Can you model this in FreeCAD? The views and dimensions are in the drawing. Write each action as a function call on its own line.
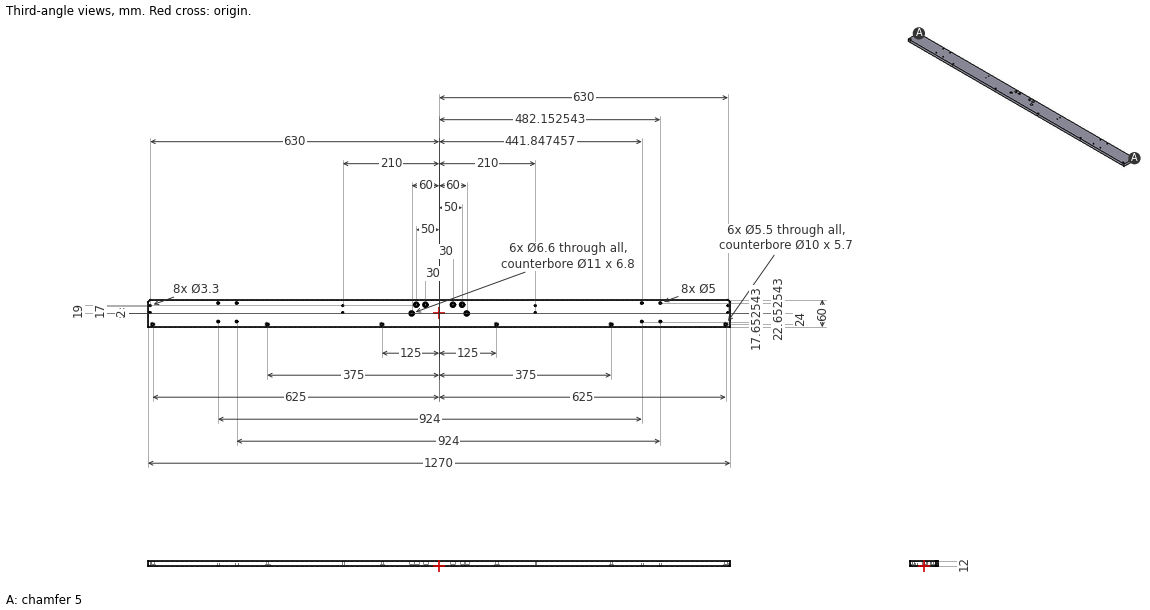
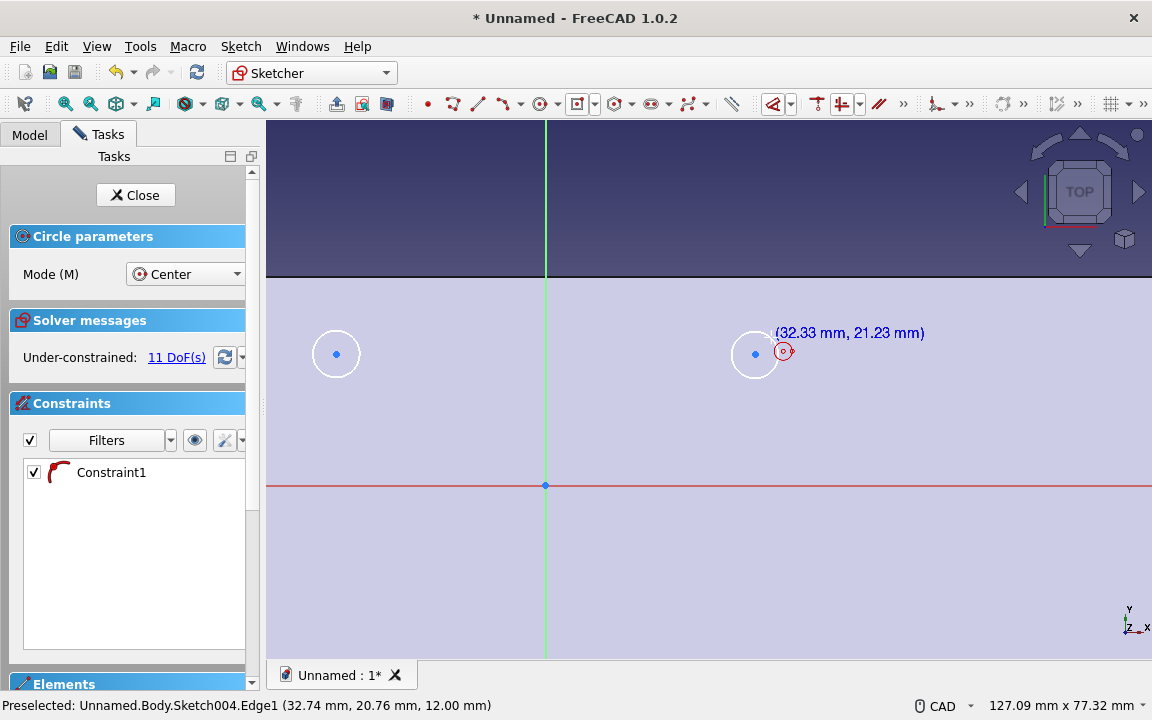
click(894, 354)
click(910, 337)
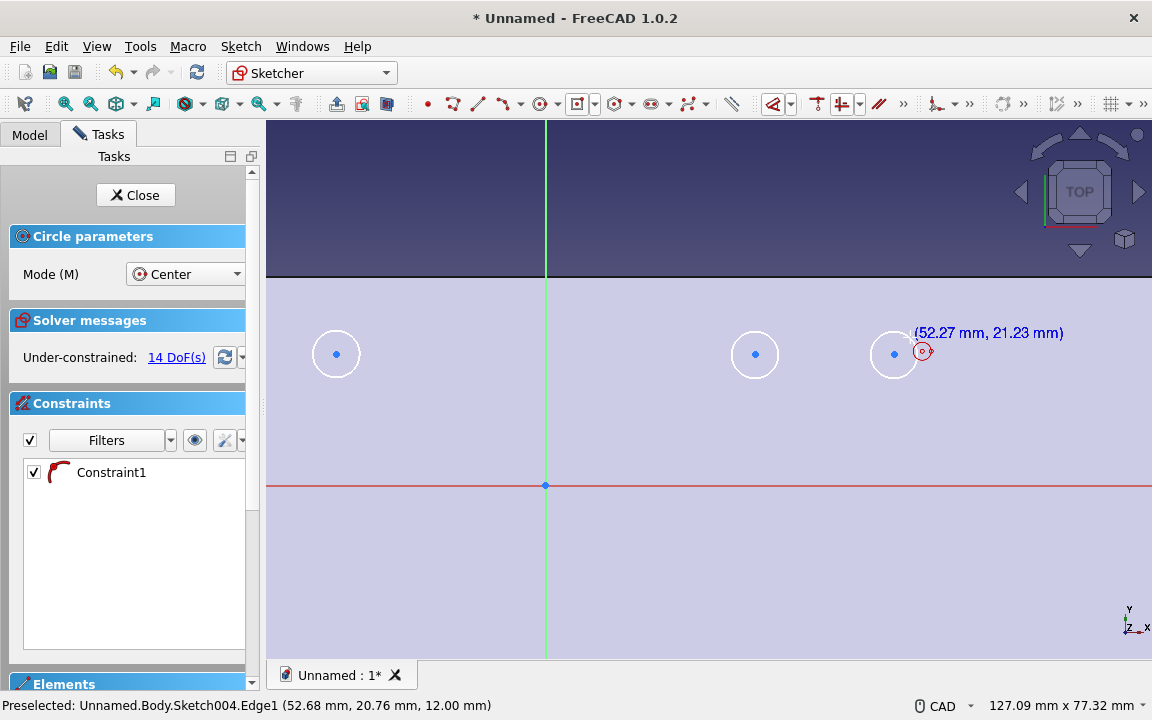
click(964, 486)
click(980, 470)
key(Escape)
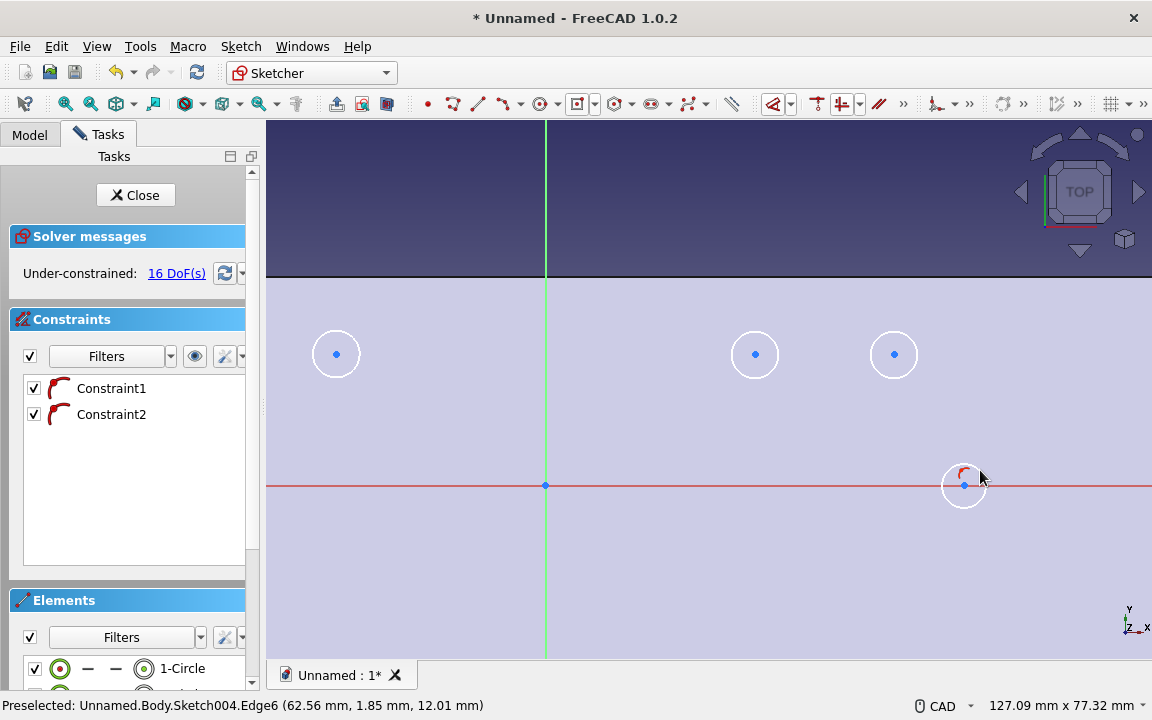
scroll(756, 353, down, 3)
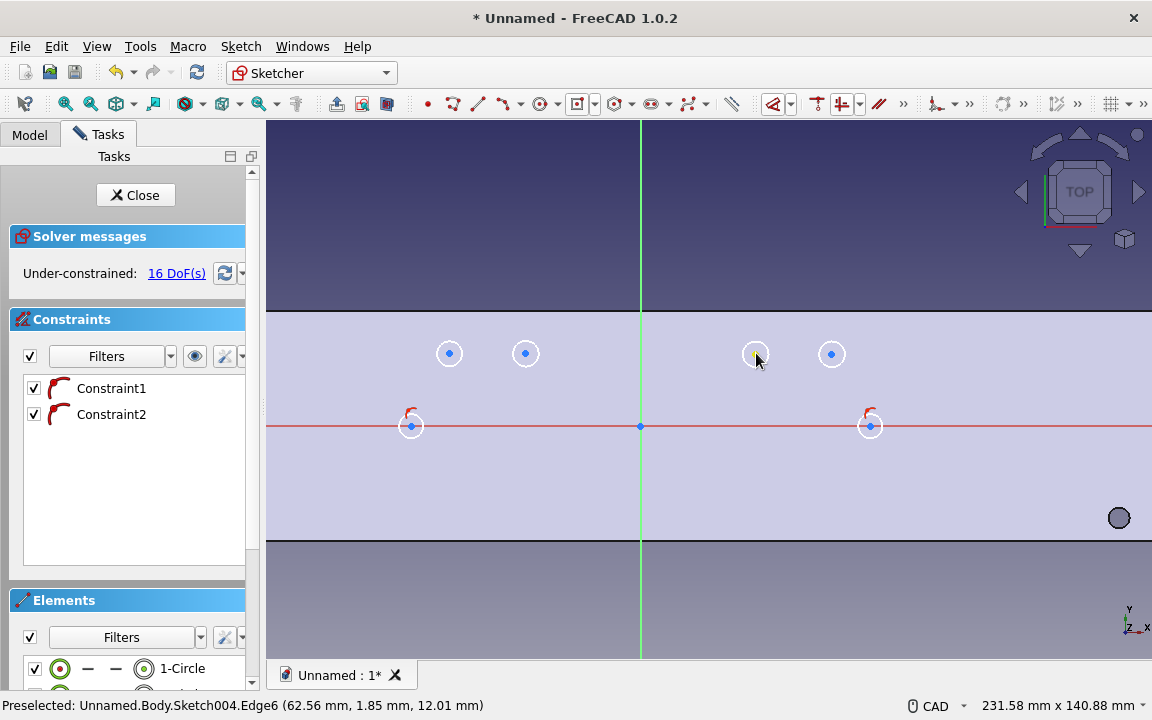
scroll(420, 418, up, 3)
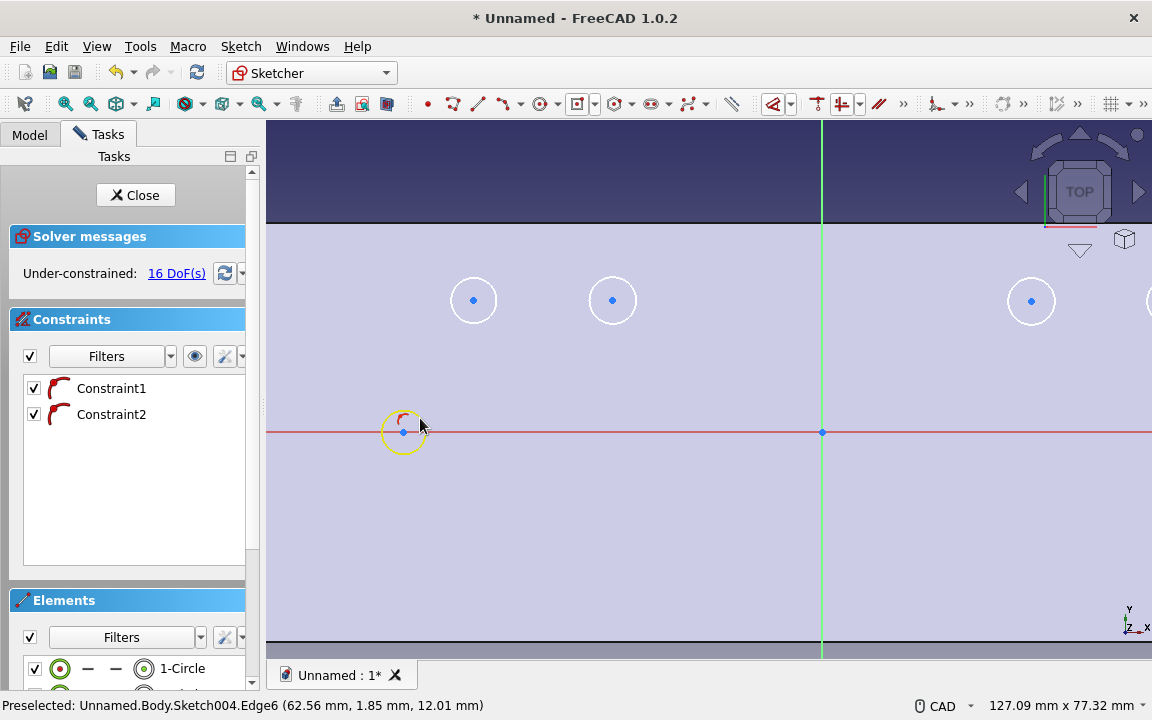
click(419, 417)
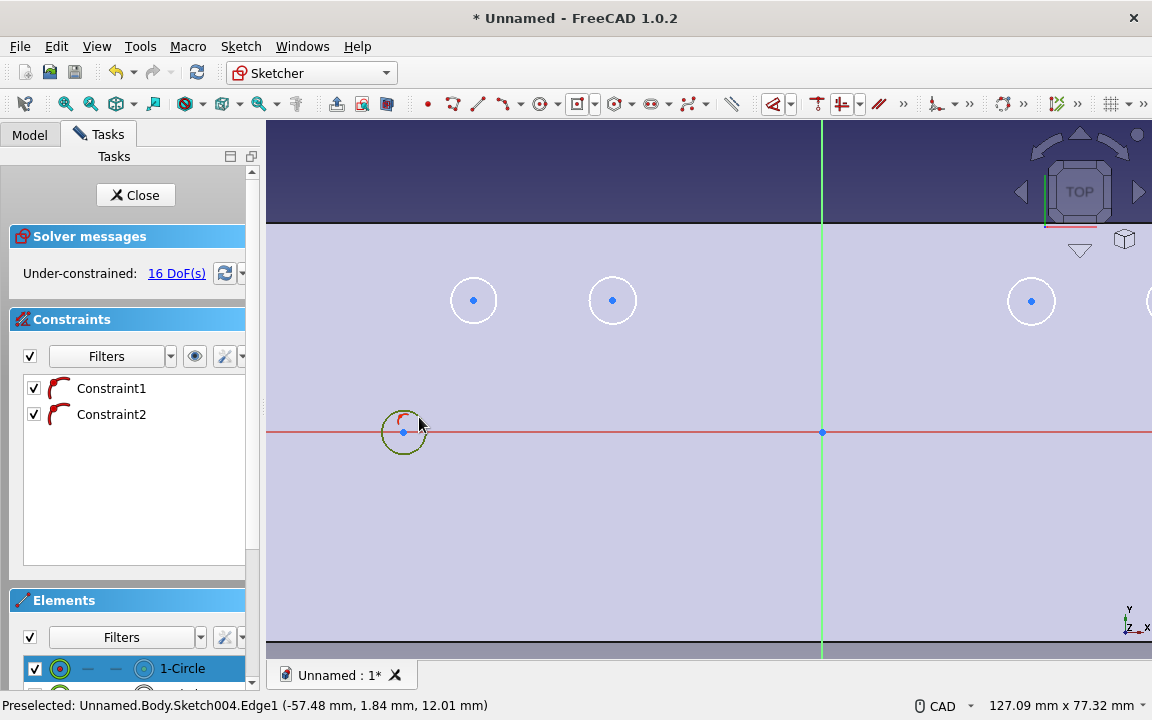
click(490, 284)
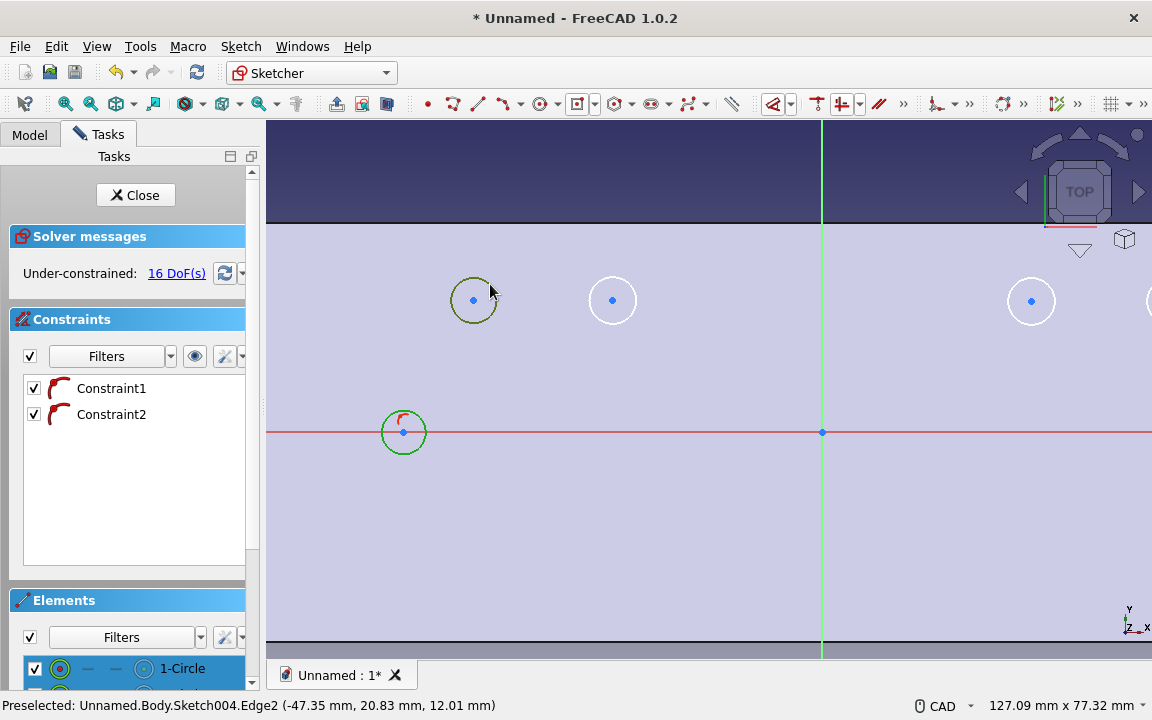
click(629, 284)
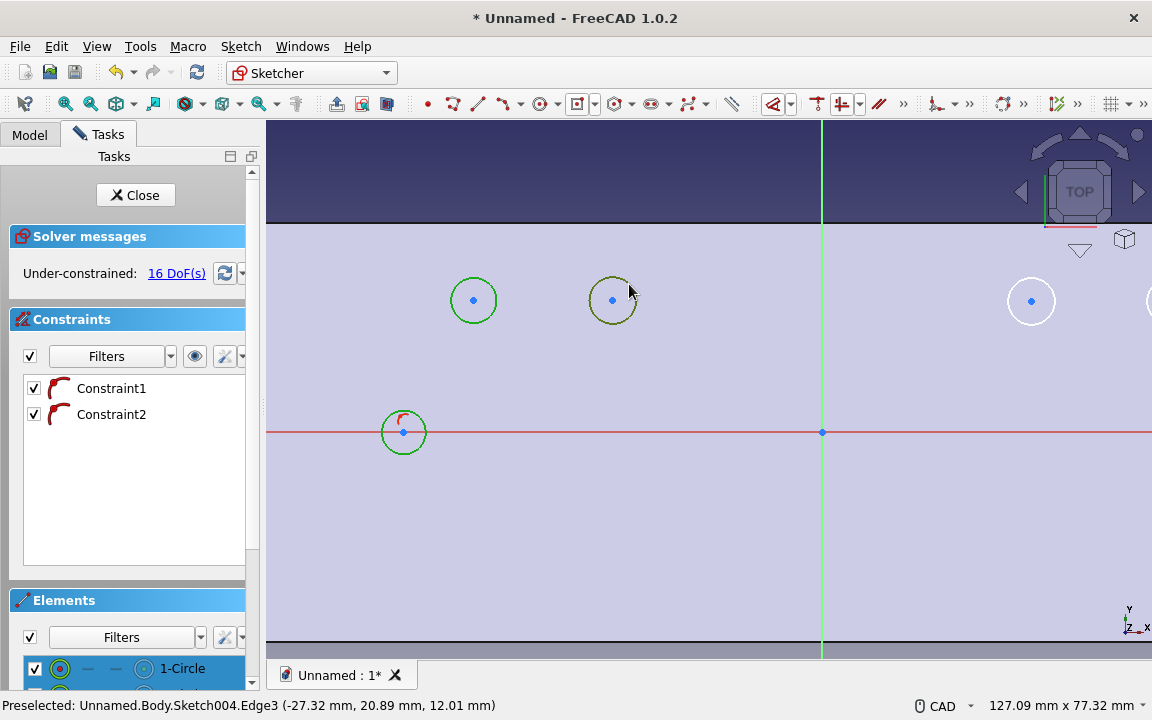
scroll(419, 418, down, 3)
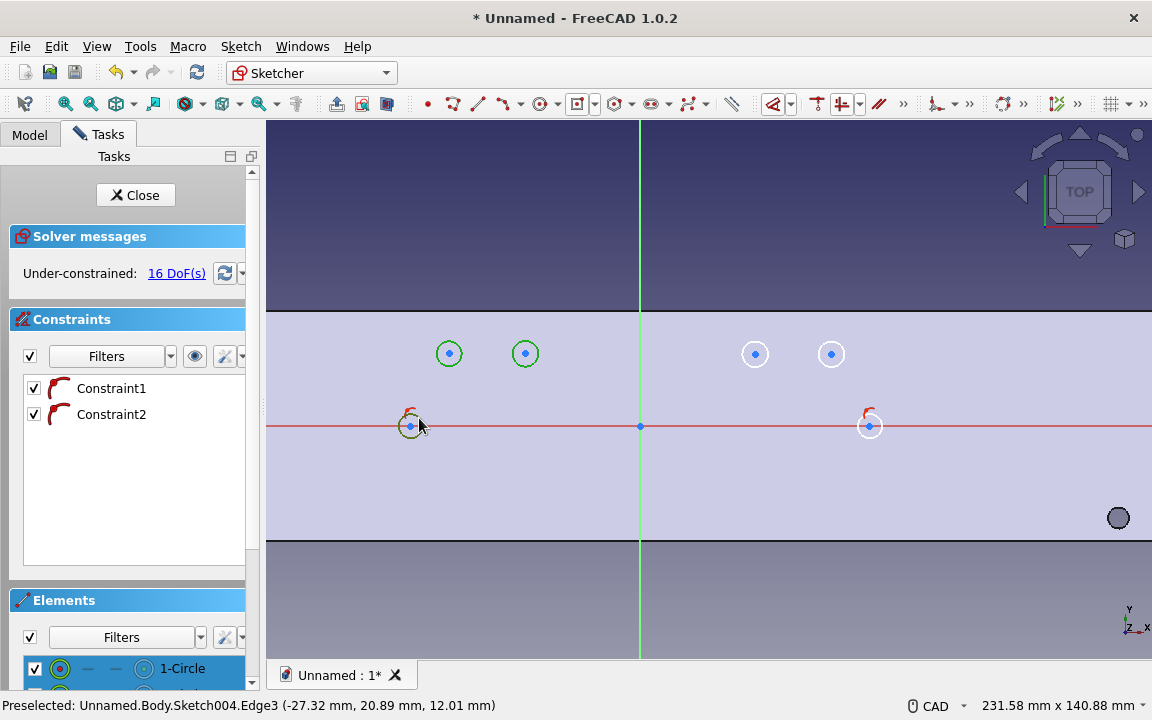
click(764, 345)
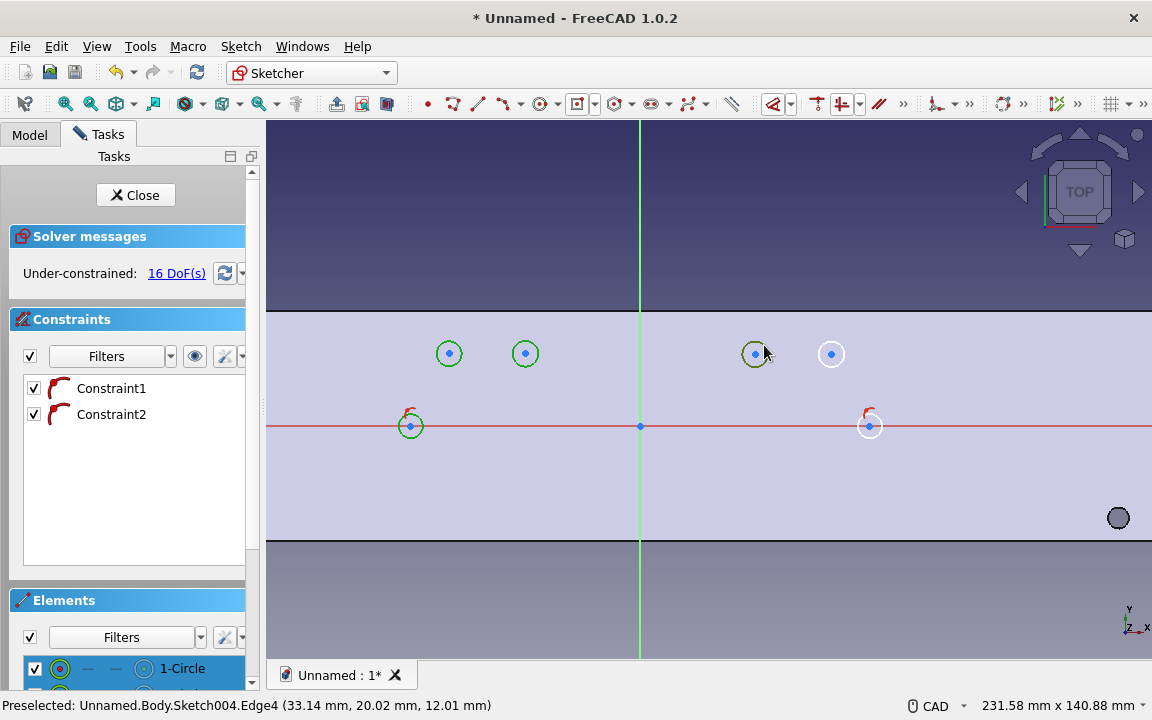
click(841, 345)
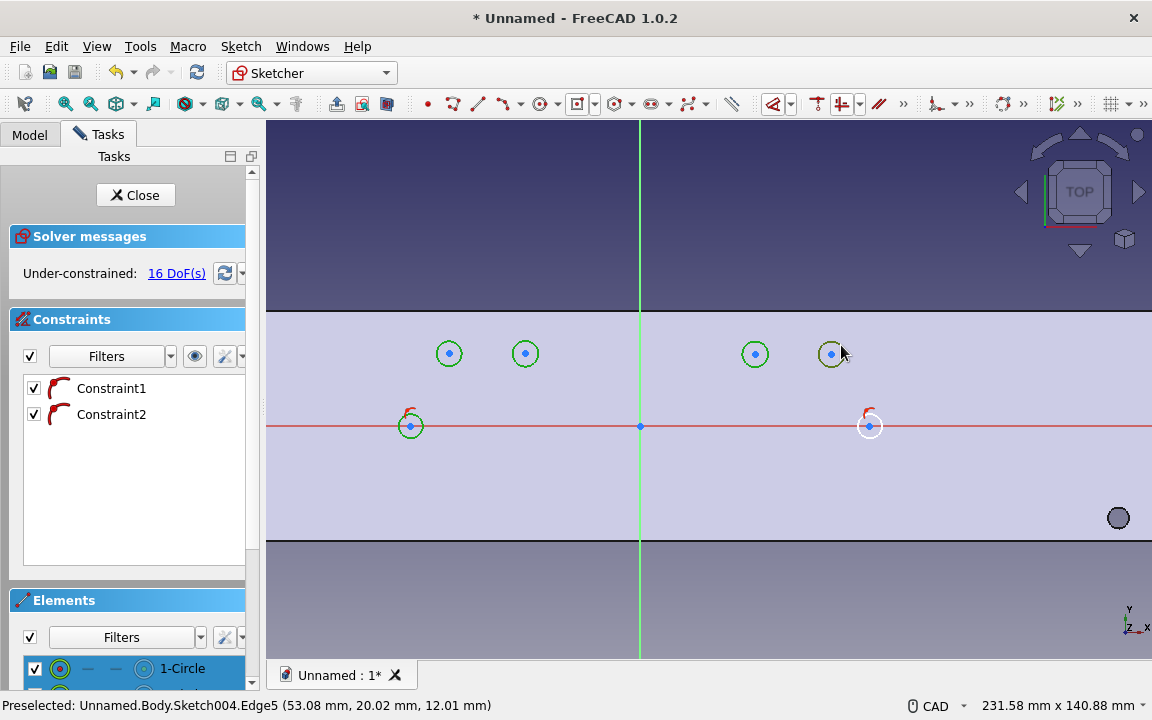
click(858, 426)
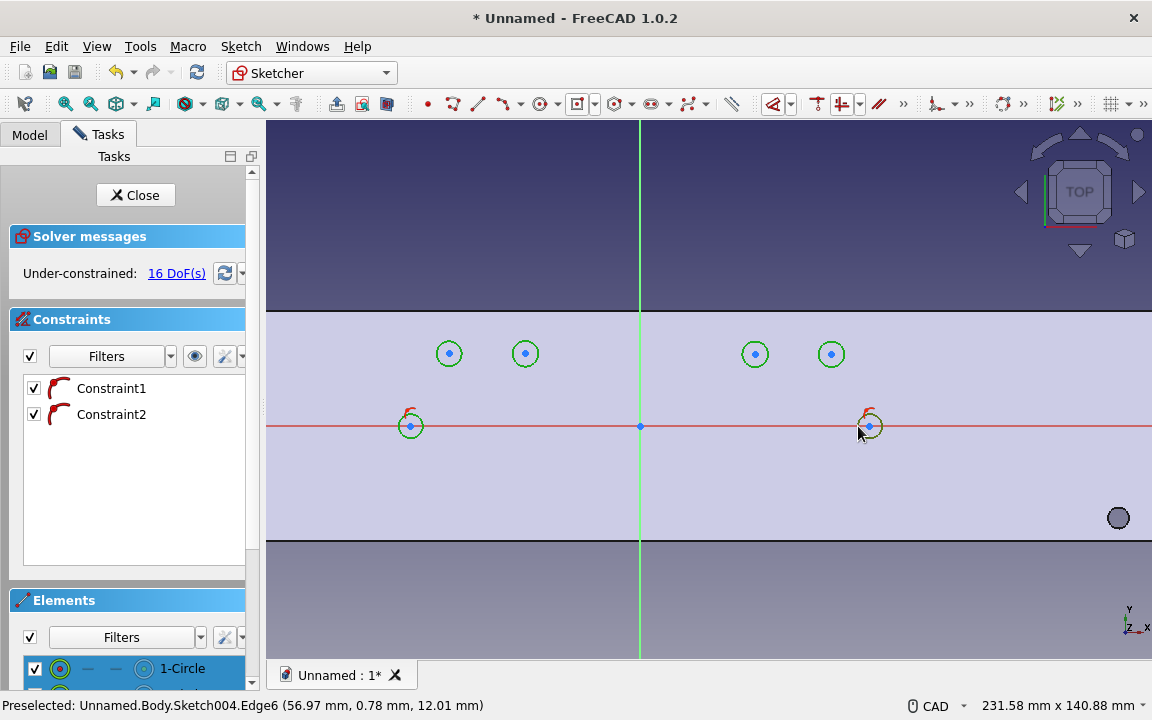
key(e)